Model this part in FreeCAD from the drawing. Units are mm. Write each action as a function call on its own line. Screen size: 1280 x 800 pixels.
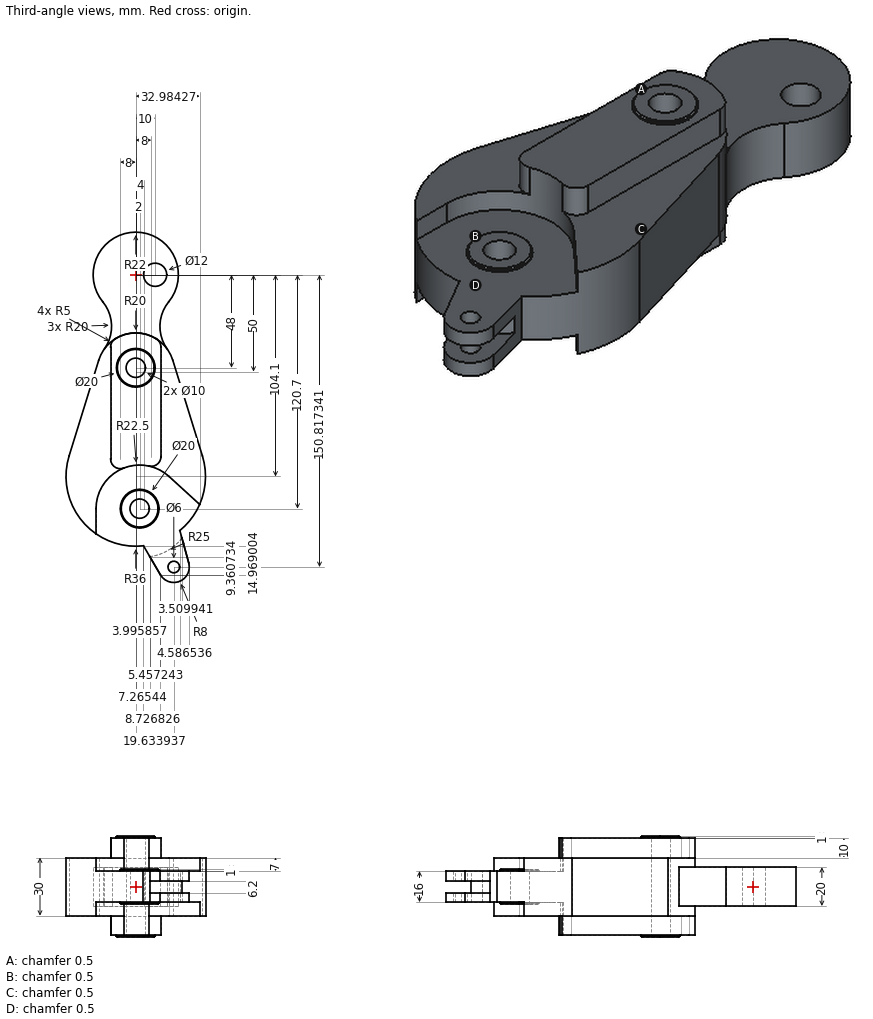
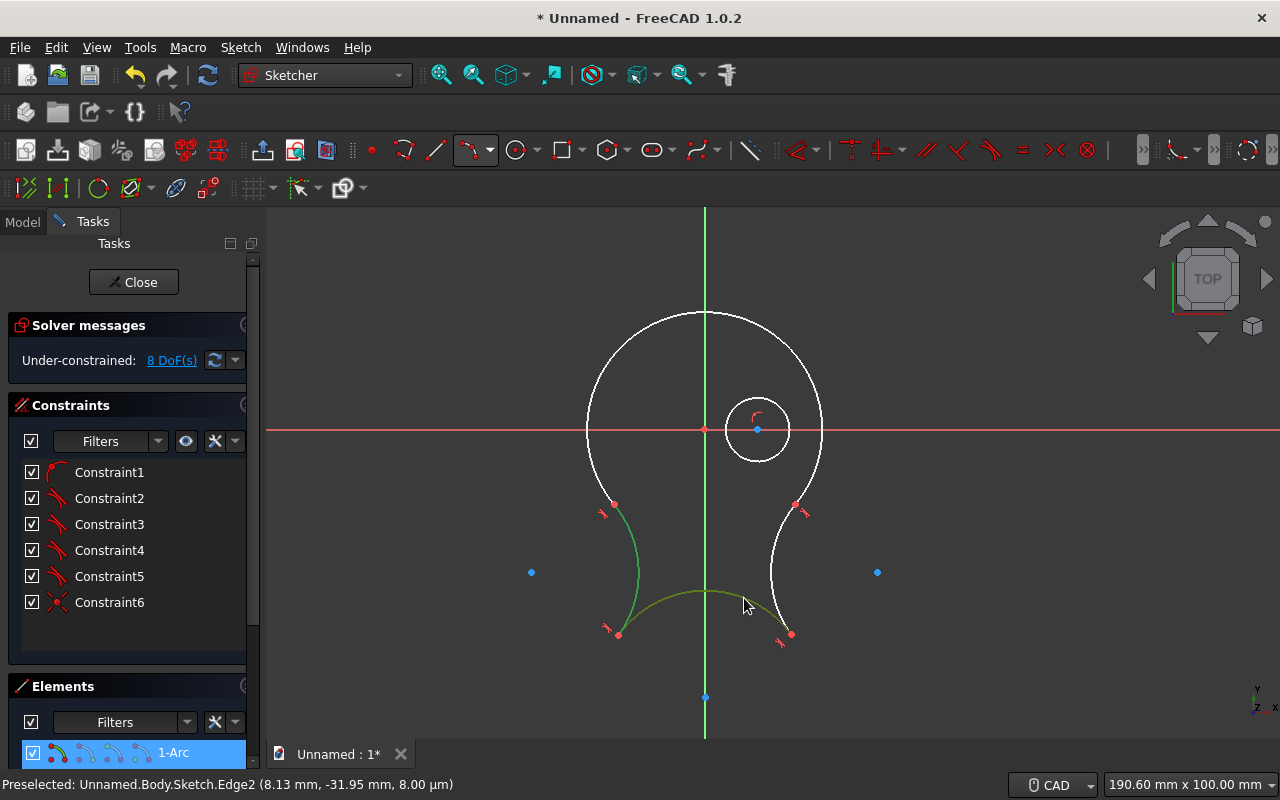
click(776, 541)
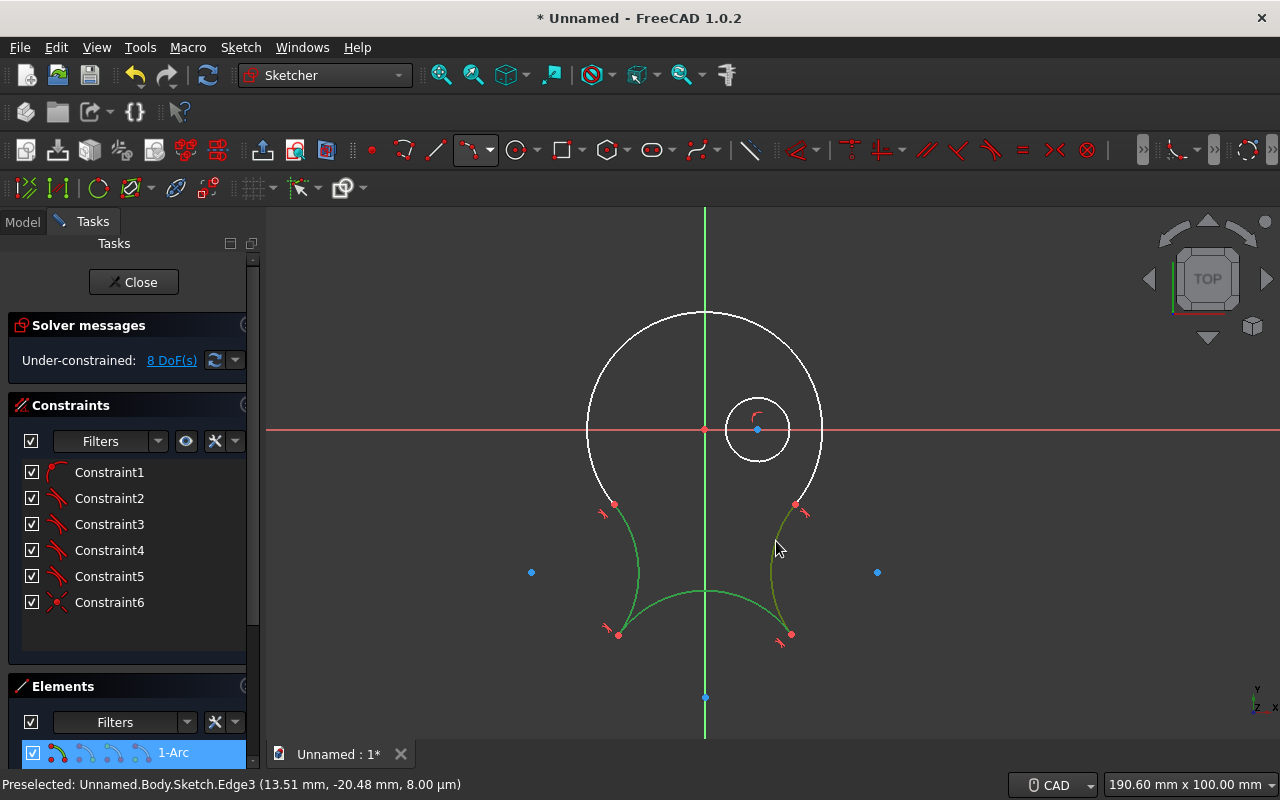
click(1024, 150)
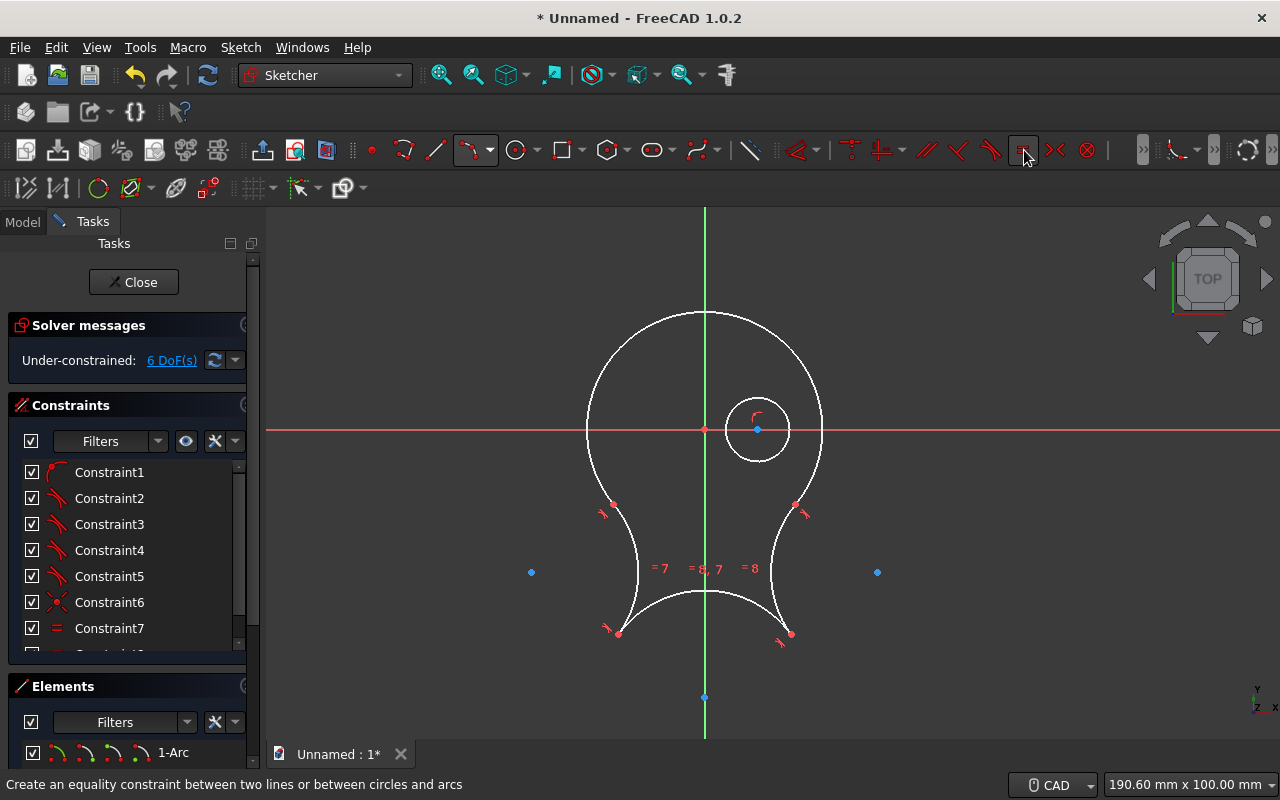
click(705, 697)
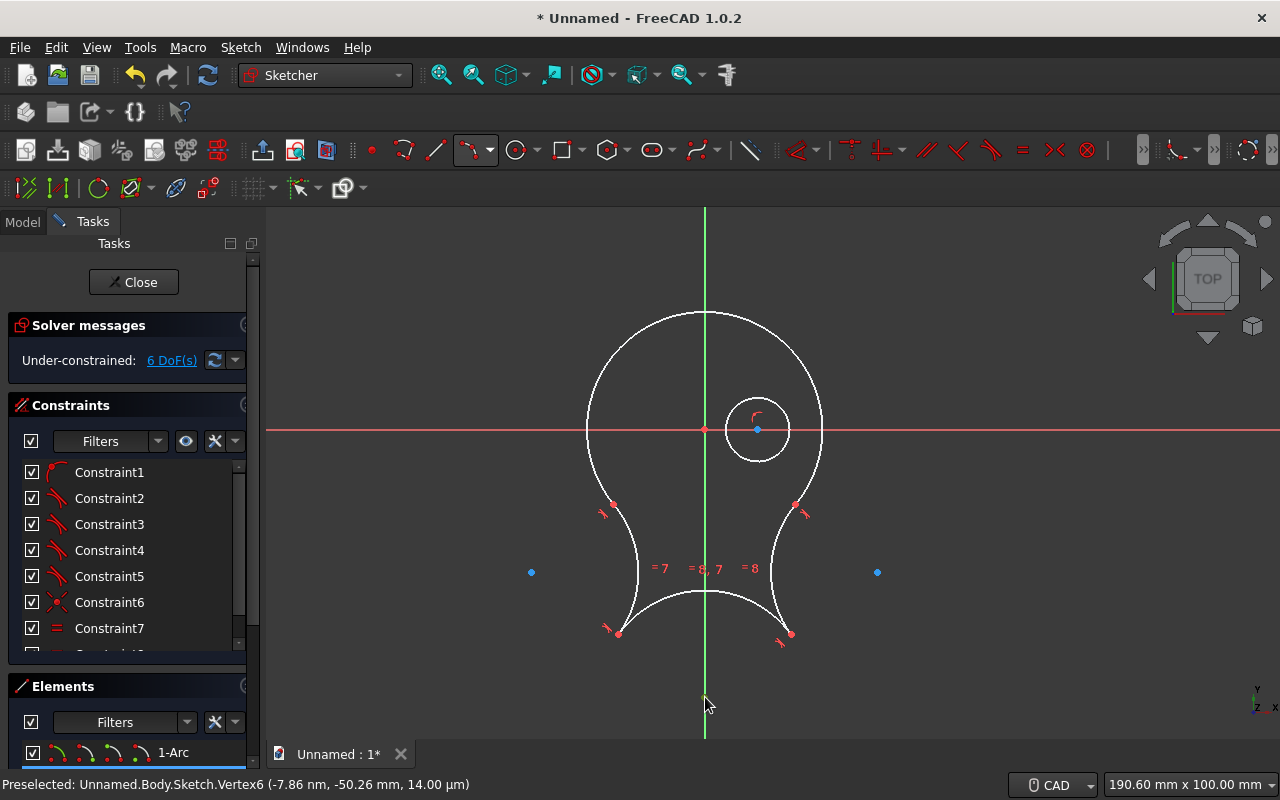
click(705, 677)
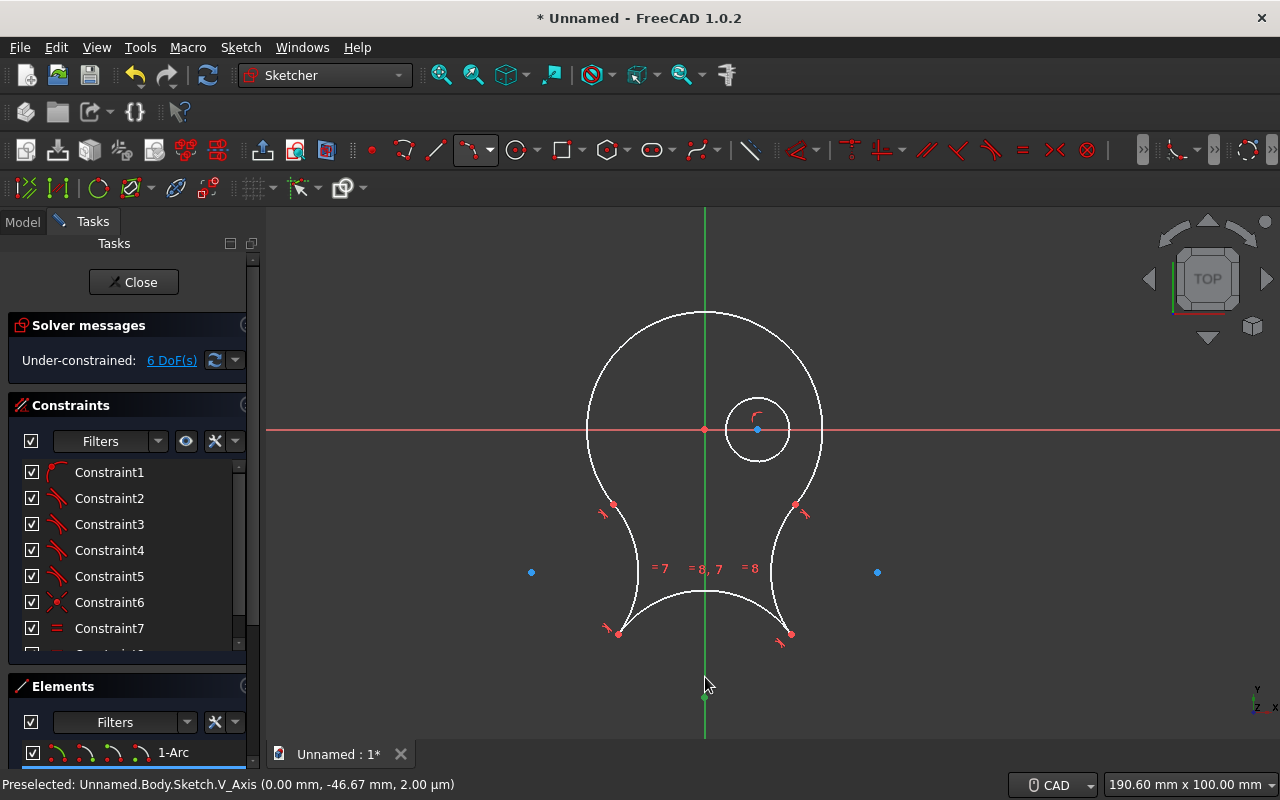
click(850, 150)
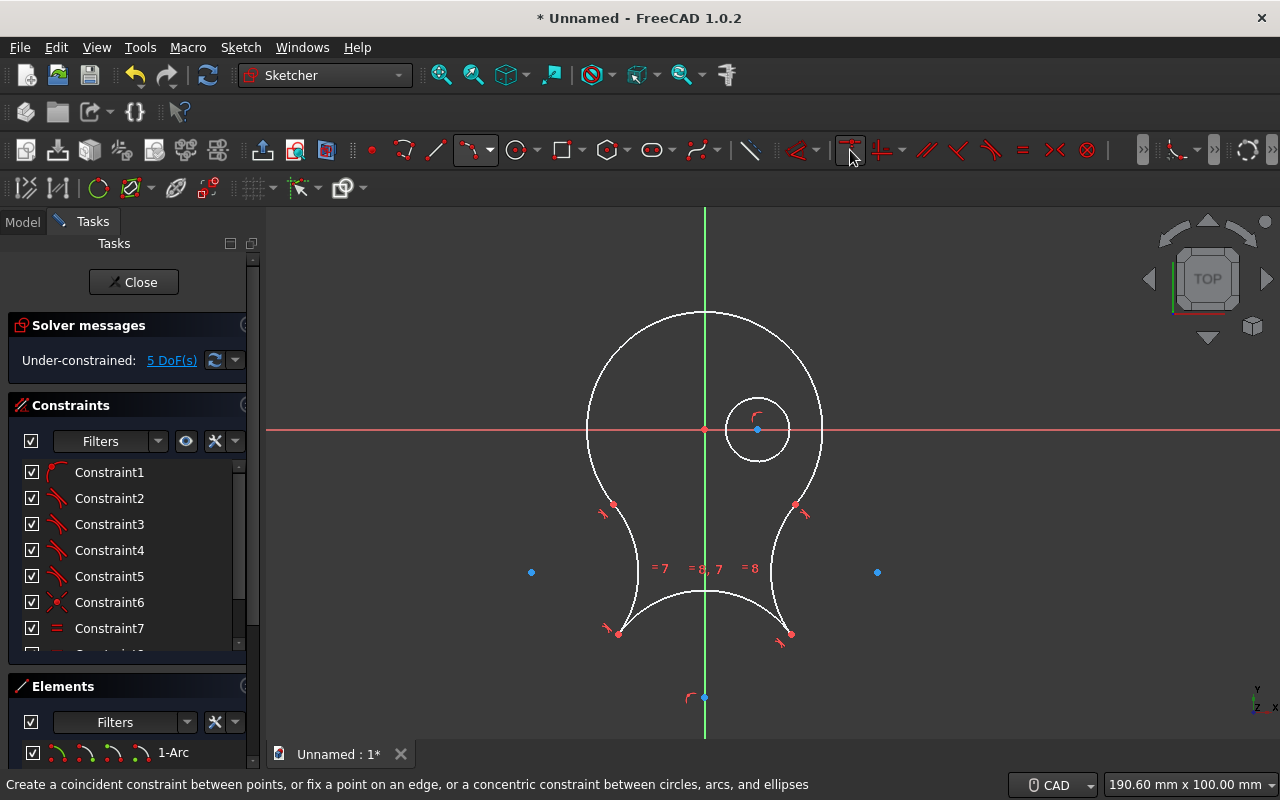
click(796, 150)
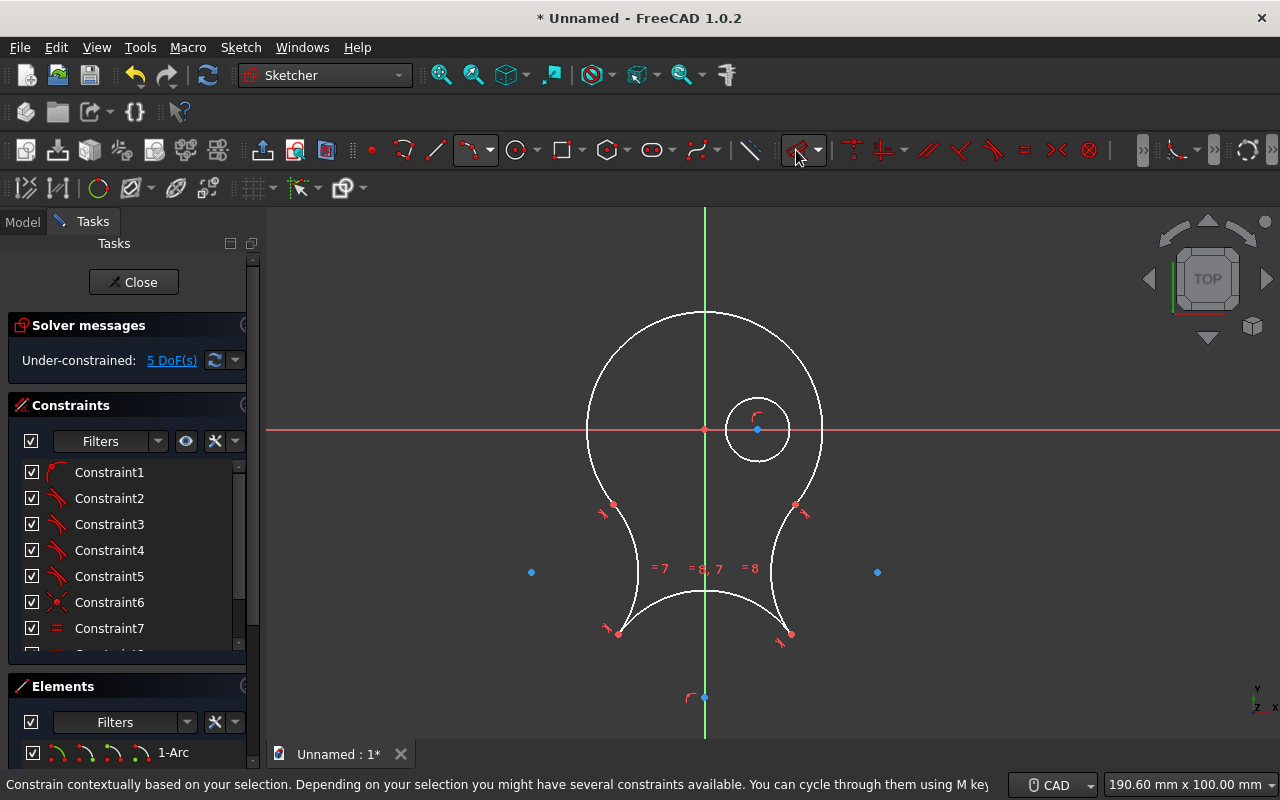
click(635, 597)
click(634, 665)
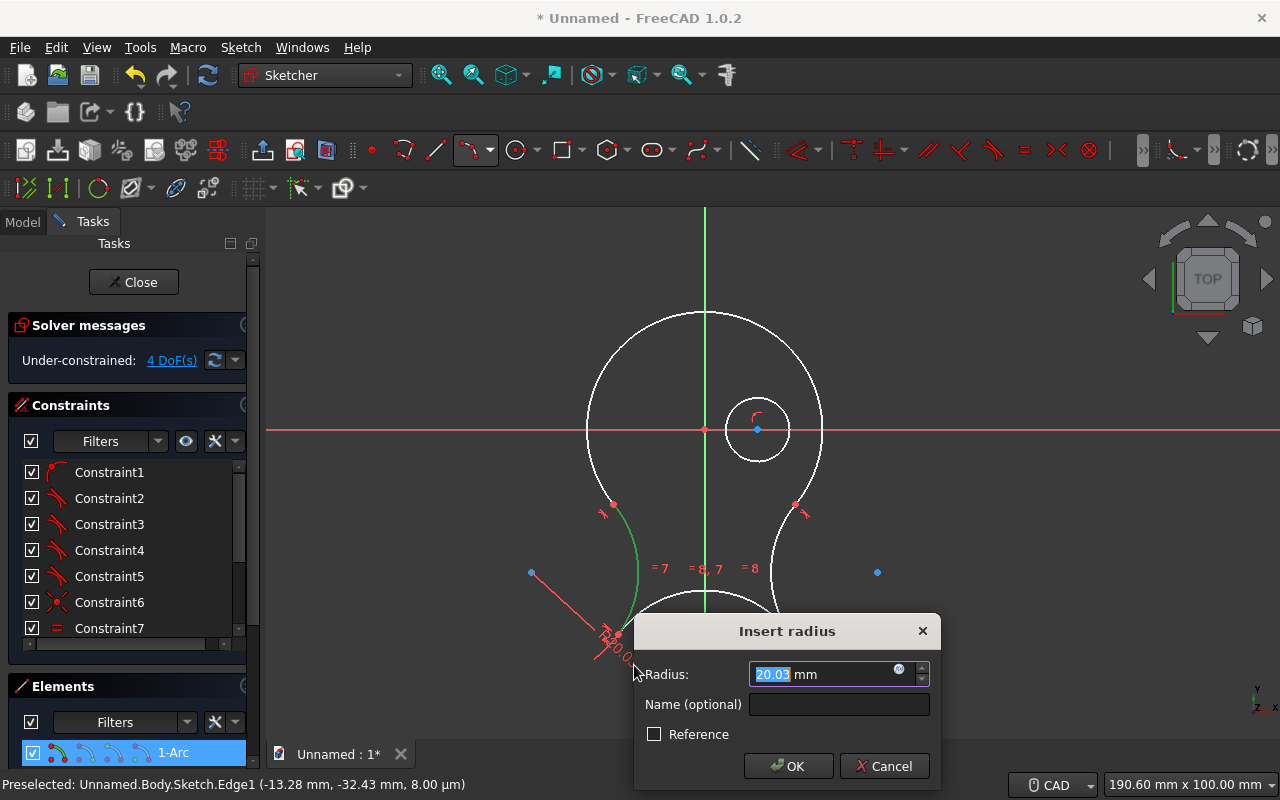
text(20)
key(Return)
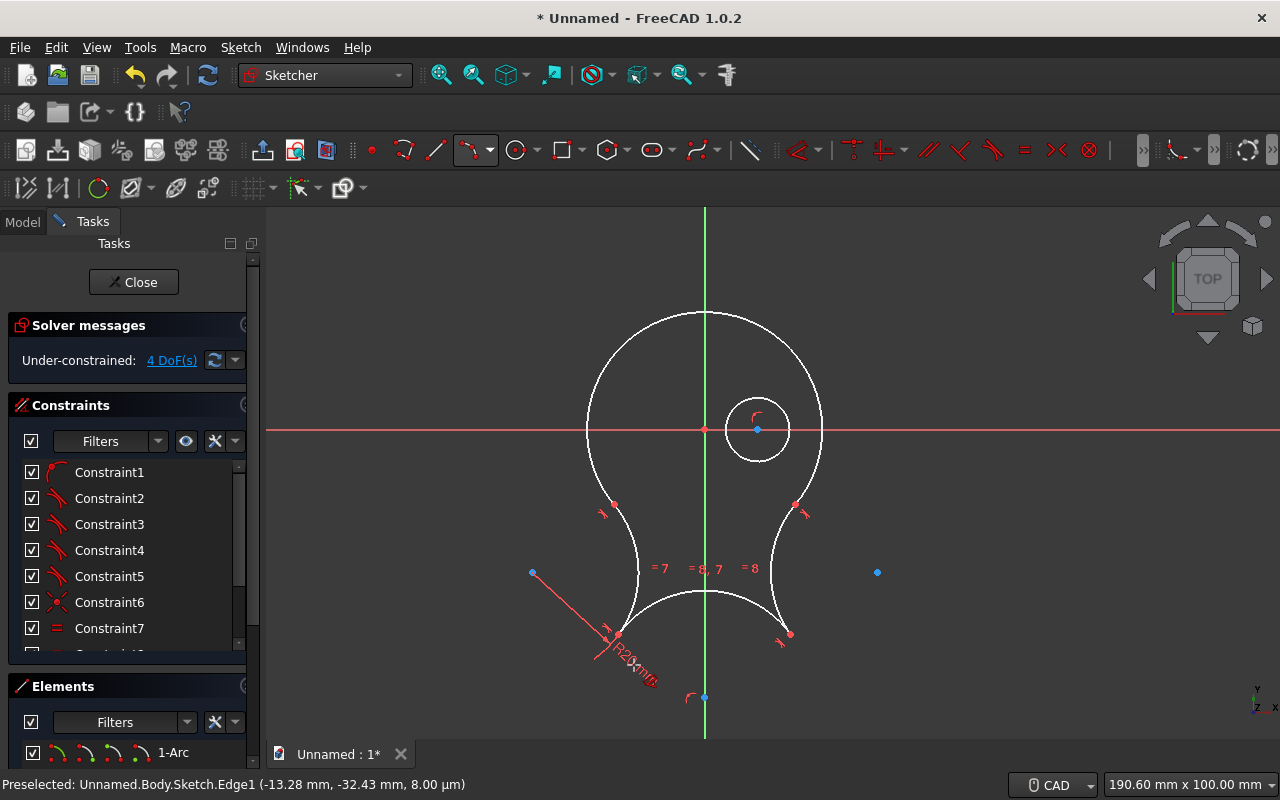
click(797, 357)
click(822, 337)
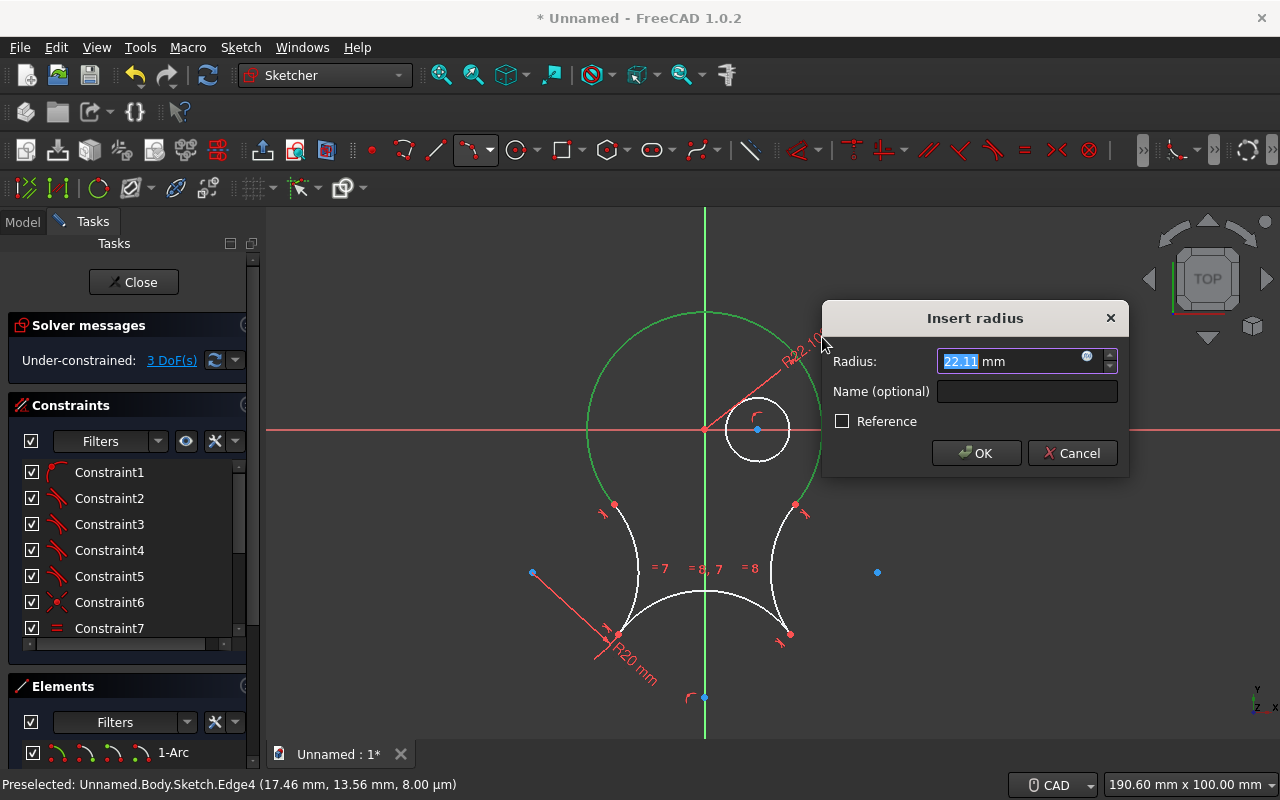
text(22)
key(Return)